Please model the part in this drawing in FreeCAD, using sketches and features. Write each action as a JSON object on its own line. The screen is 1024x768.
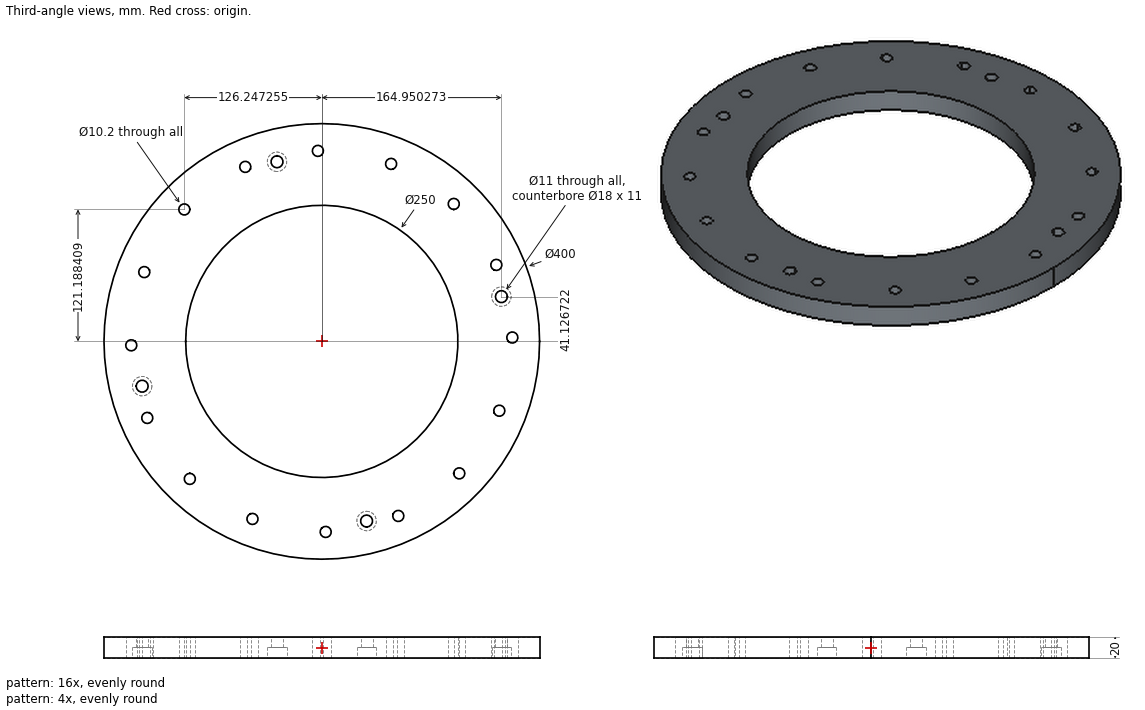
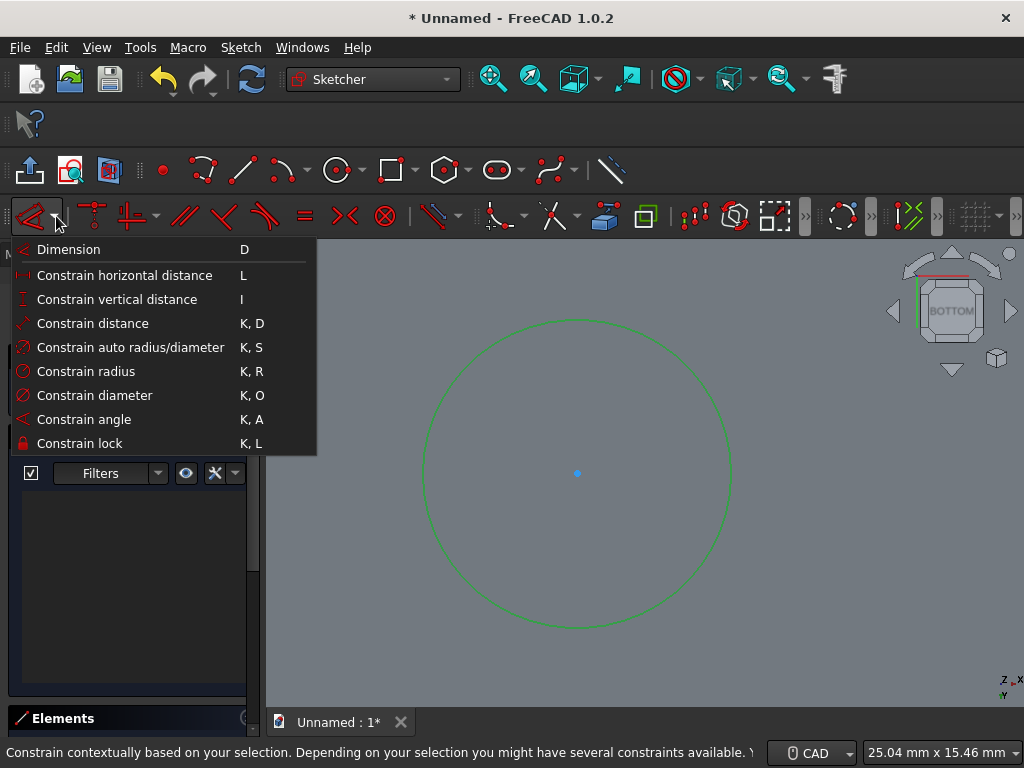
{"action": "left_click", "coordinate": [164, 395]}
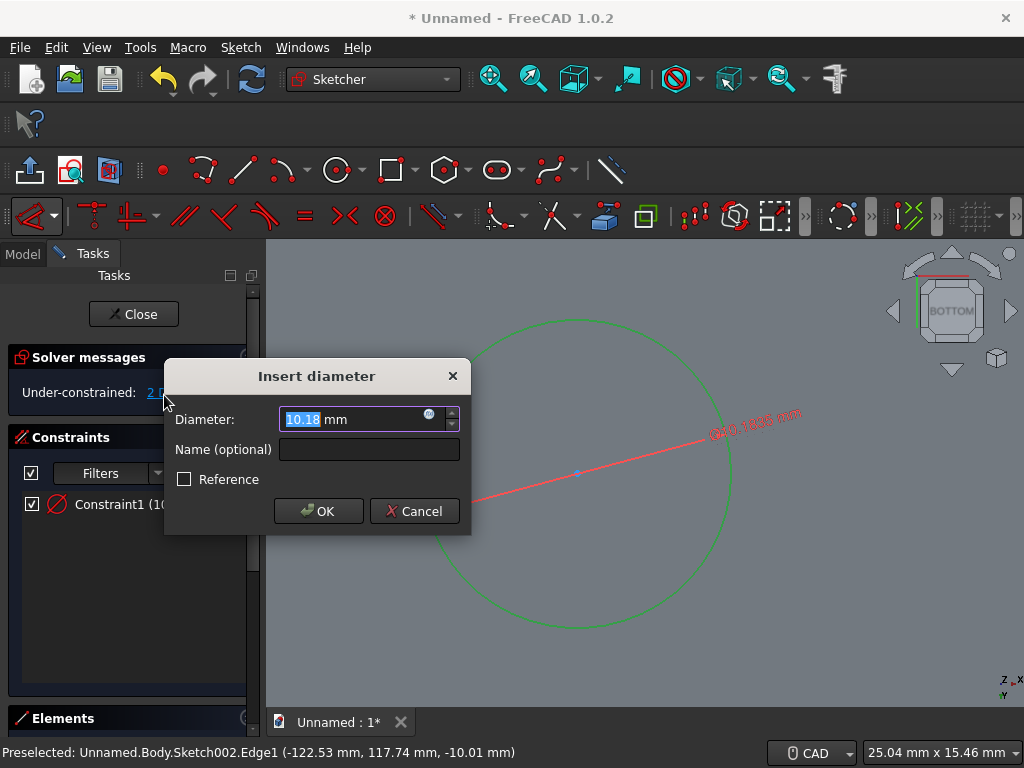
{"action": "type", "text": "10.2"}
{"action": "key", "text": "Return"}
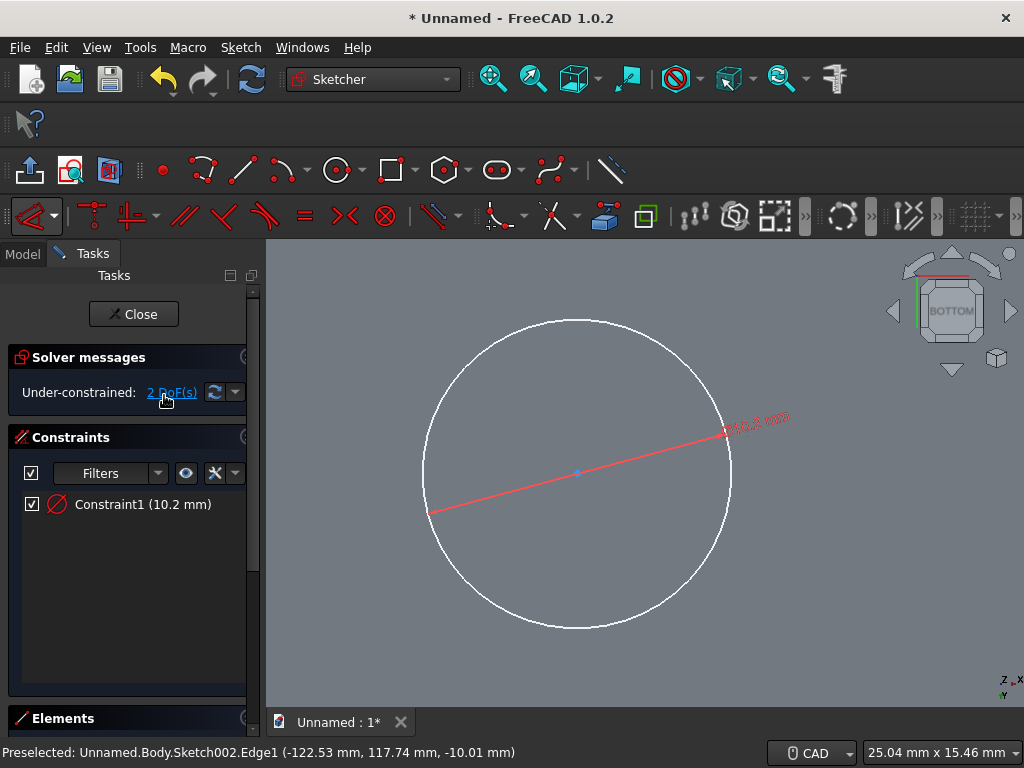
{"action": "left_click", "coordinate": [577, 474]}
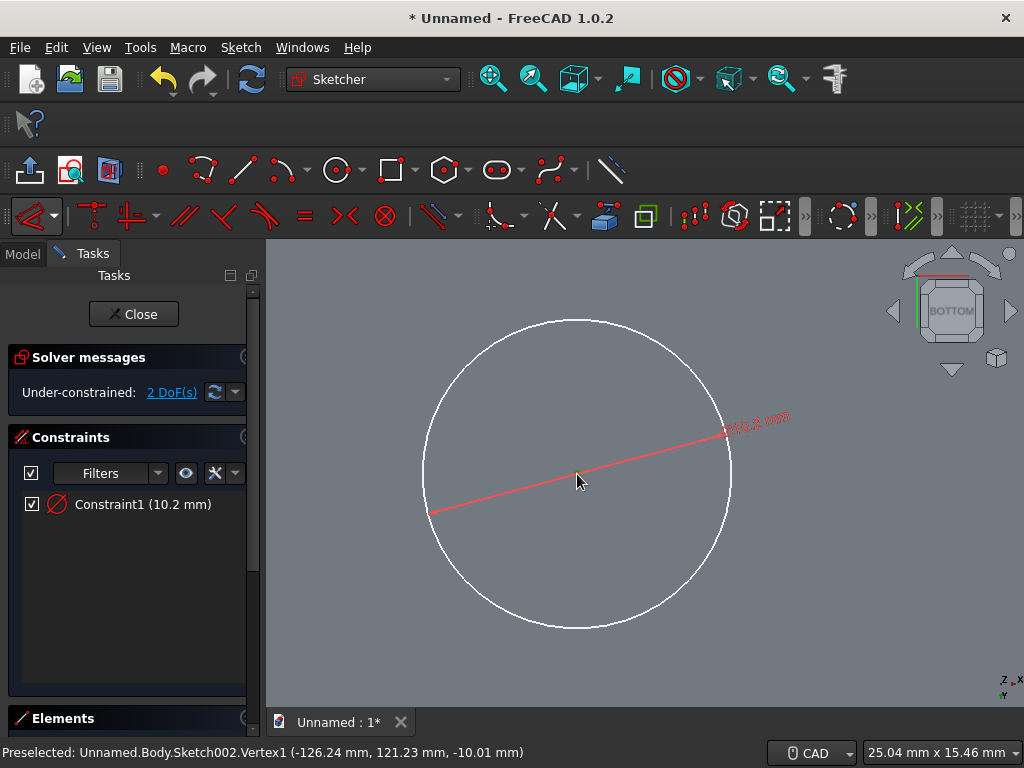
{"action": "key", "text": "l"}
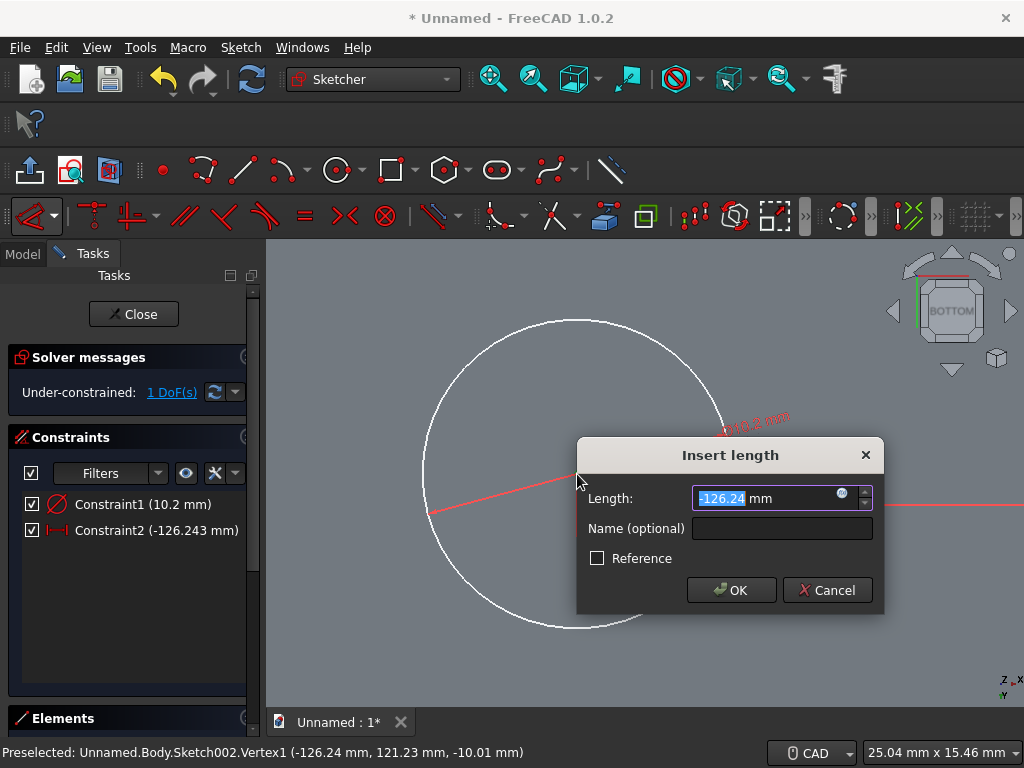
{"action": "type", "text": "-126.247255"}
{"action": "key", "text": "Return"}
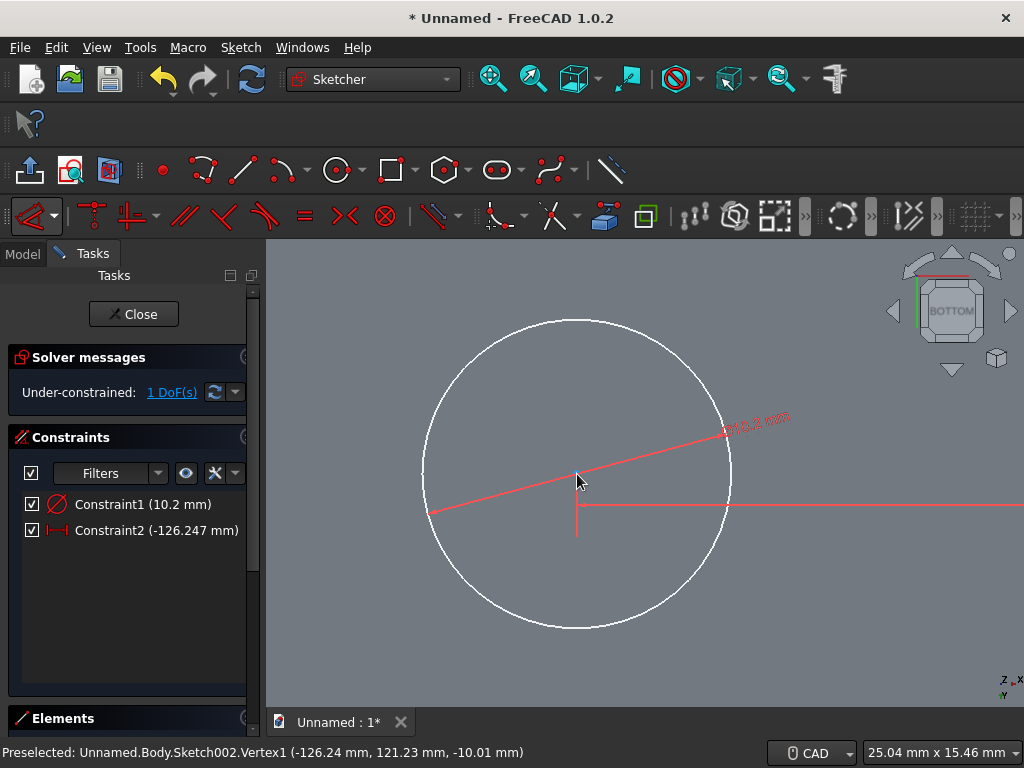
{"action": "left_click", "coordinate": [577, 474]}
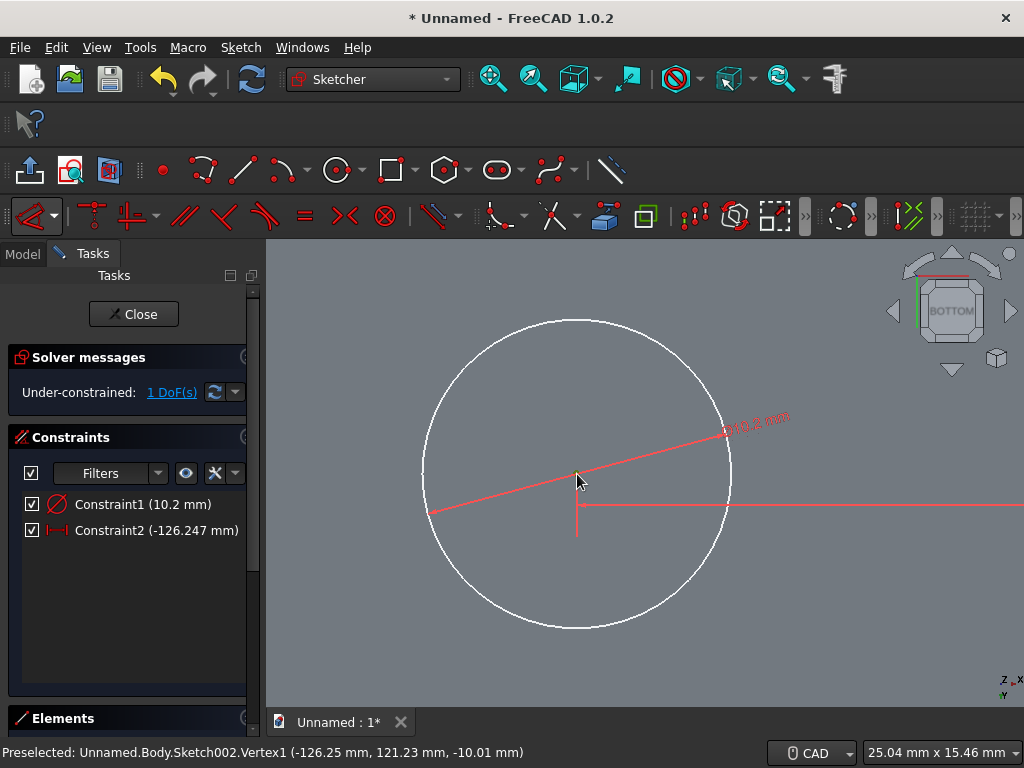
{"action": "left_click", "coordinate": [56, 216]}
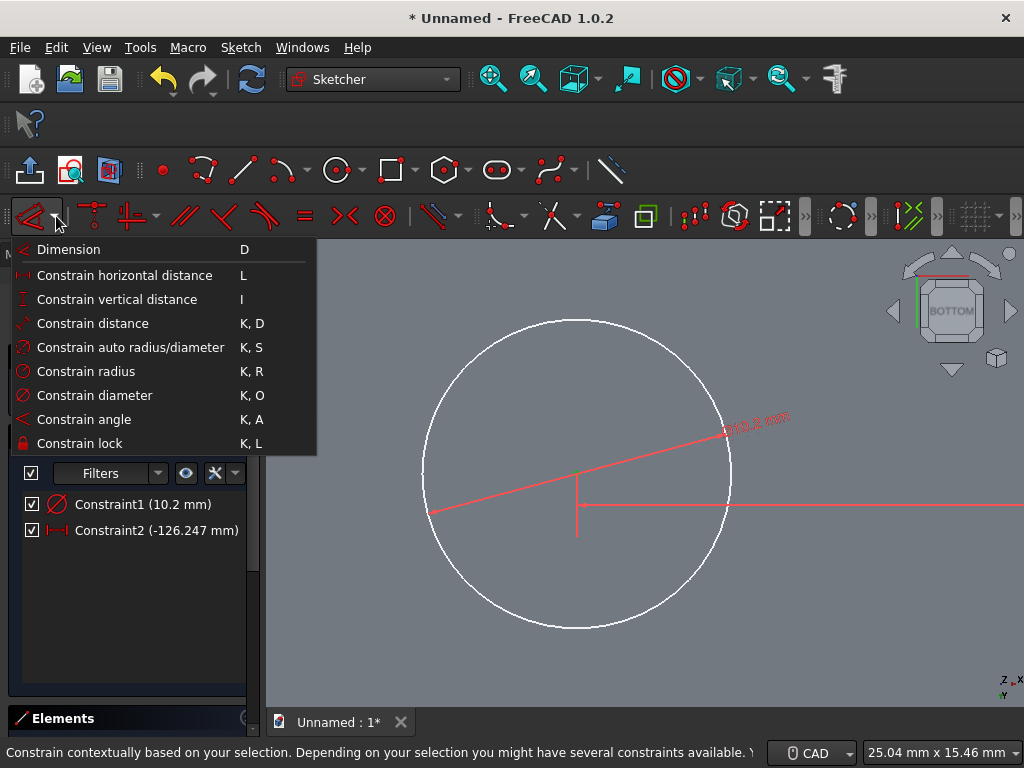
{"action": "left_click", "coordinate": [164, 299]}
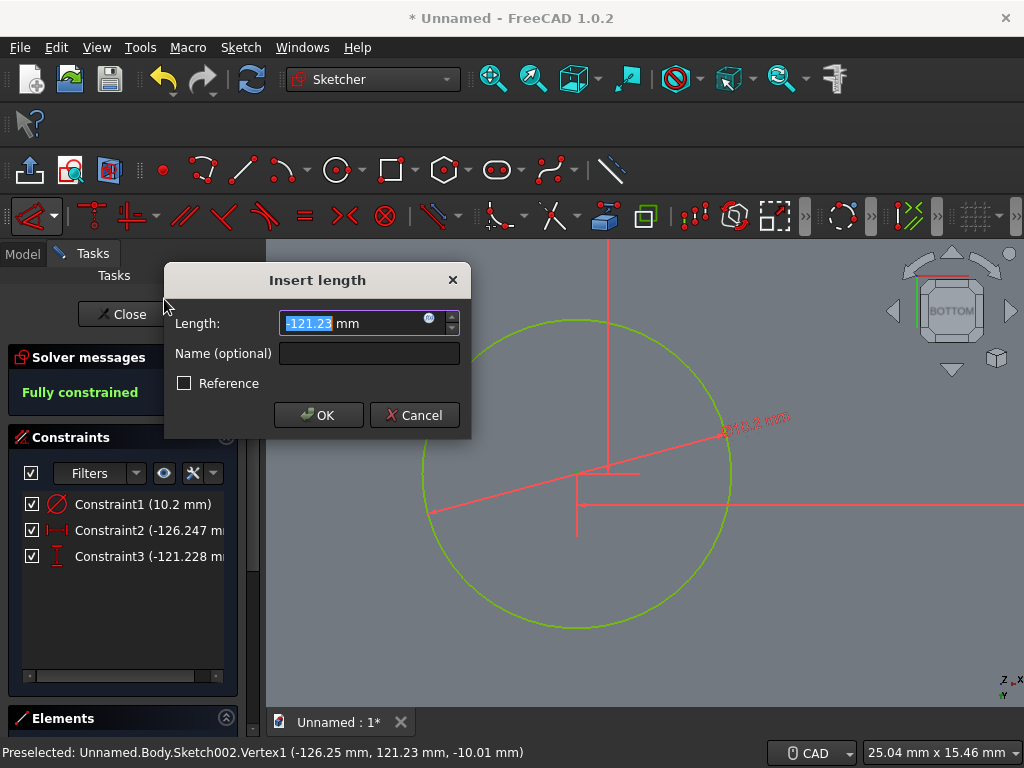
{"action": "type", "text": "-121.188409"}
{"action": "key", "text": "Return"}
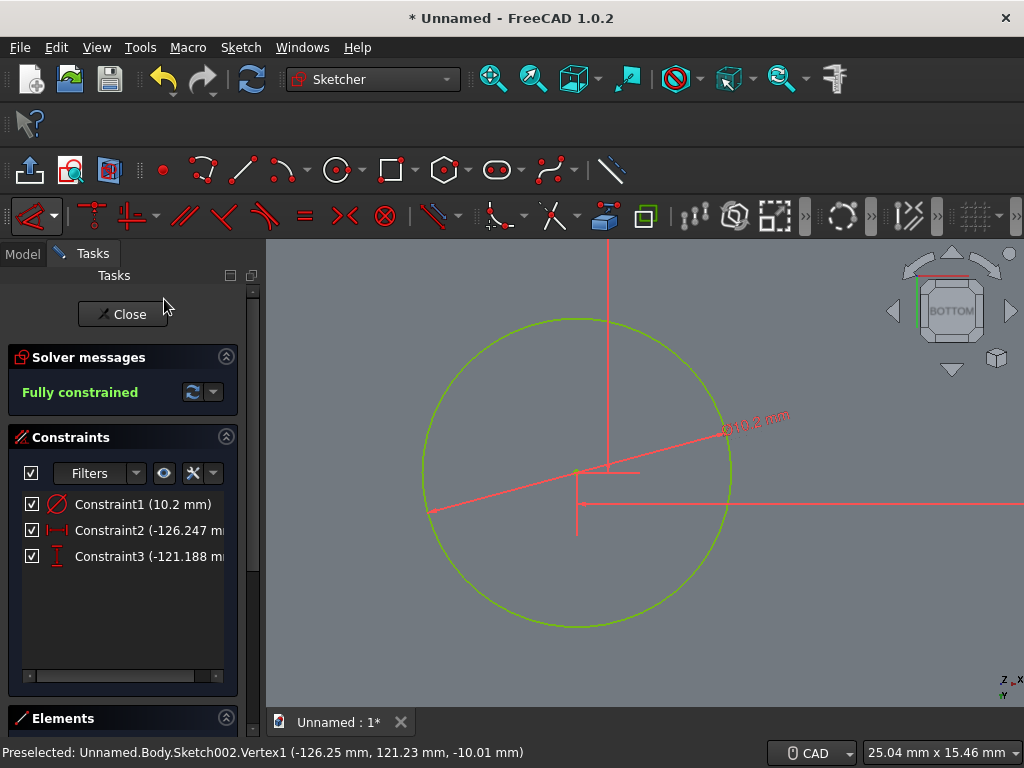
{"action": "left_click", "coordinate": [123, 314]}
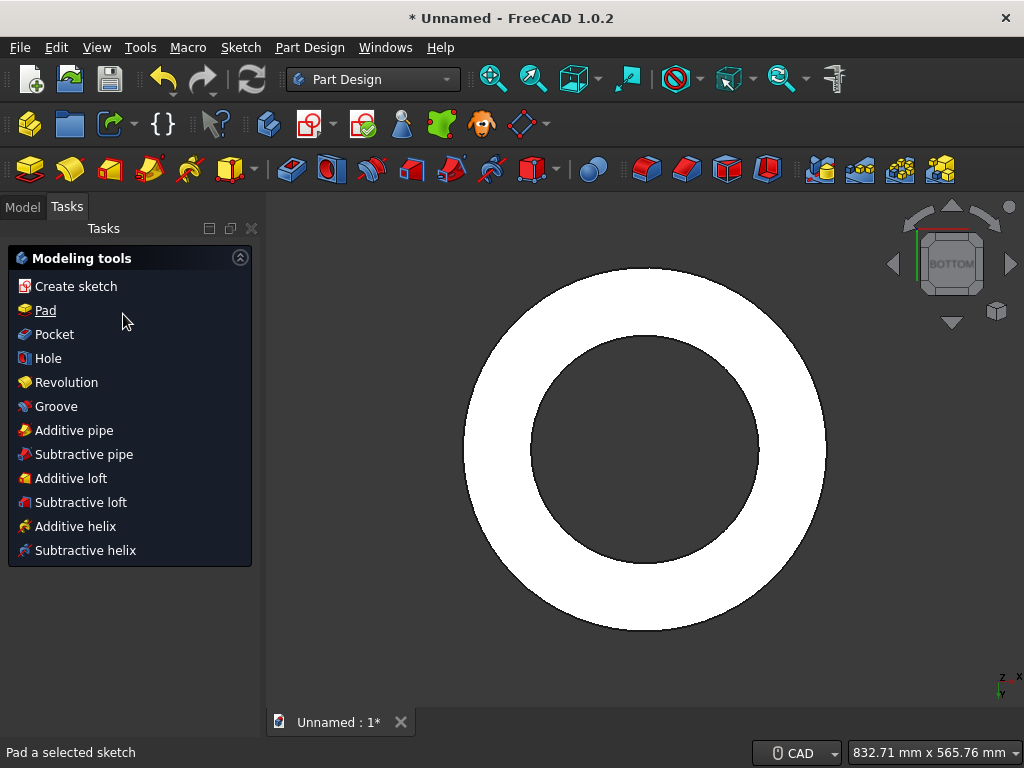
{"action": "left_click", "coordinate": [332, 170]}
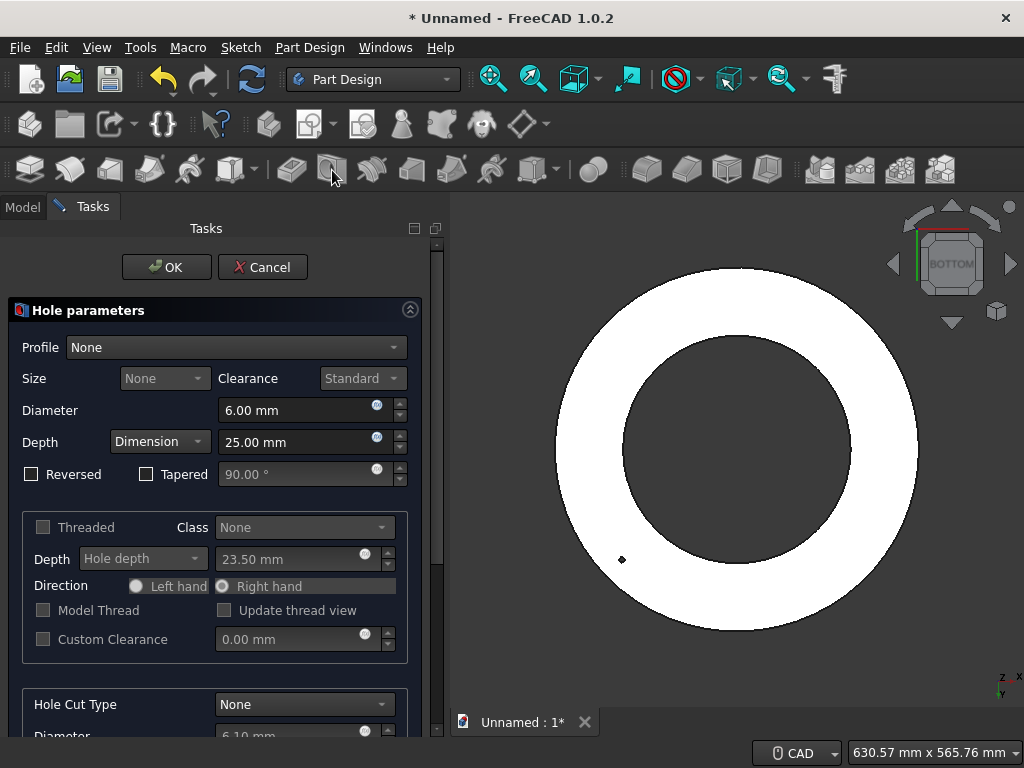
{"action": "triple_click", "coordinate": [305, 410]}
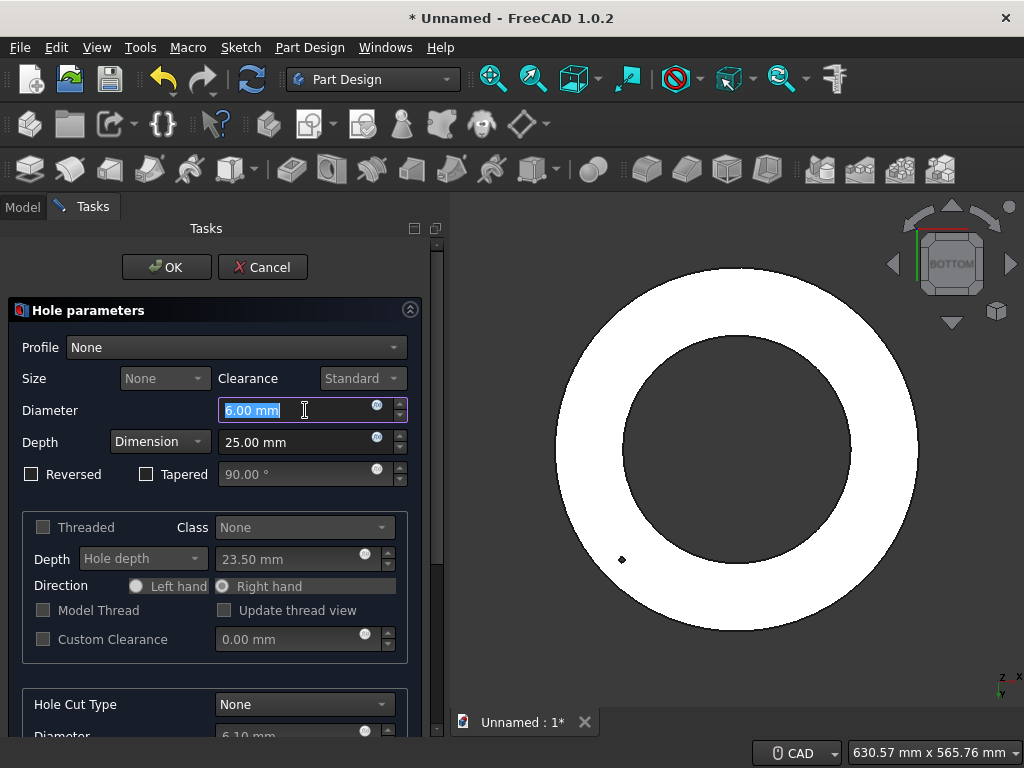
{"action": "type", "text": "10.2"}
{"action": "key", "text": "Tab"}